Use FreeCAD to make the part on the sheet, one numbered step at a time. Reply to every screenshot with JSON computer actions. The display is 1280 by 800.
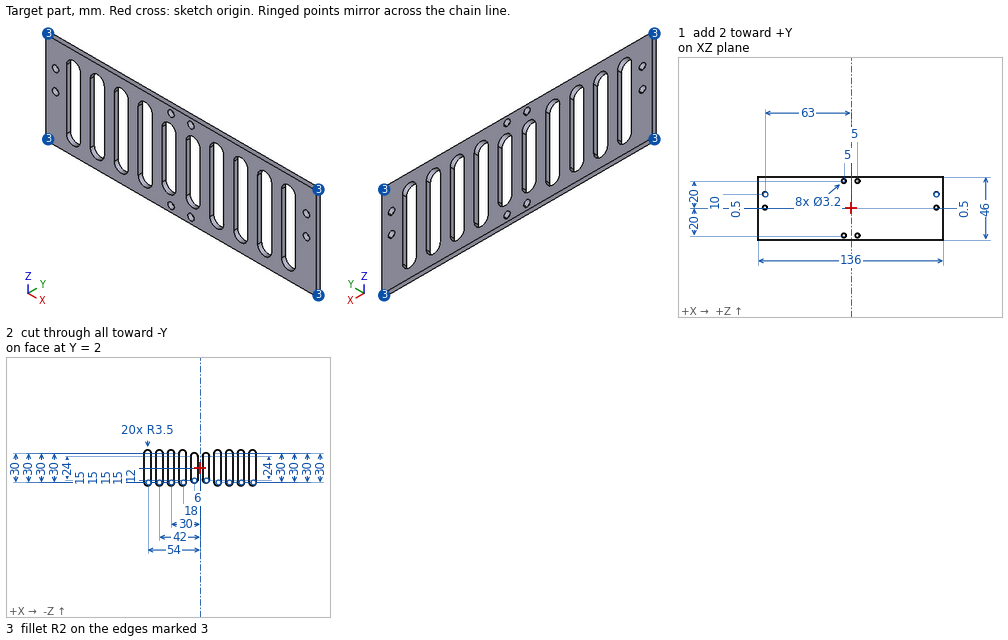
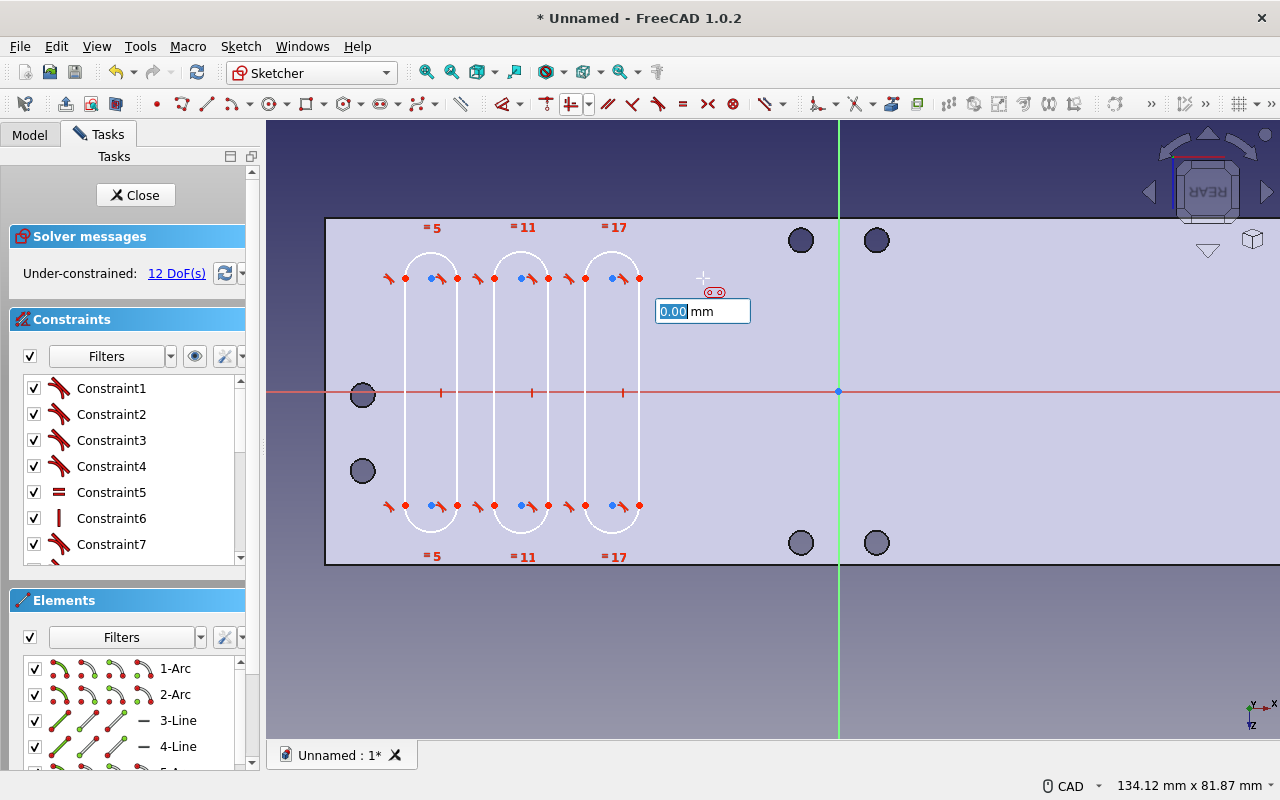
{"action": "left_click", "coordinate": [729, 426]}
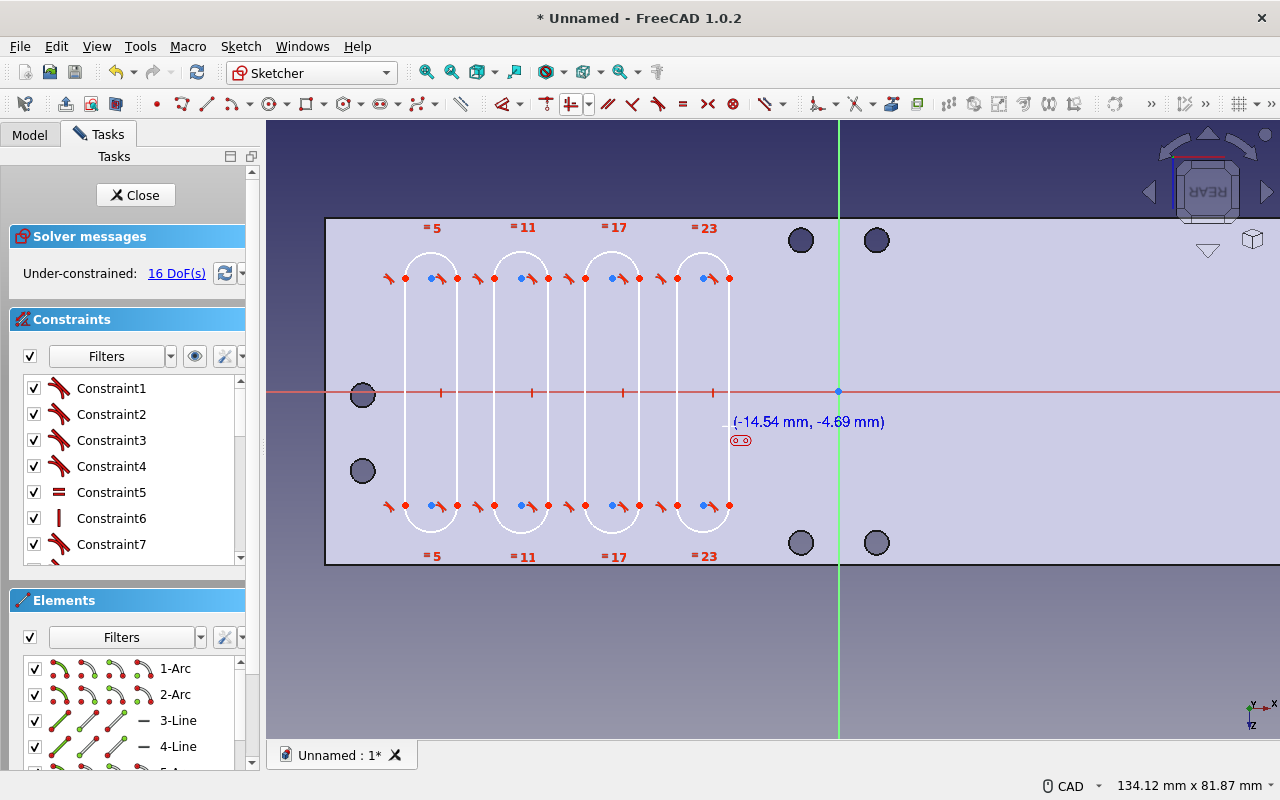
{"action": "left_click", "coordinate": [794, 482]}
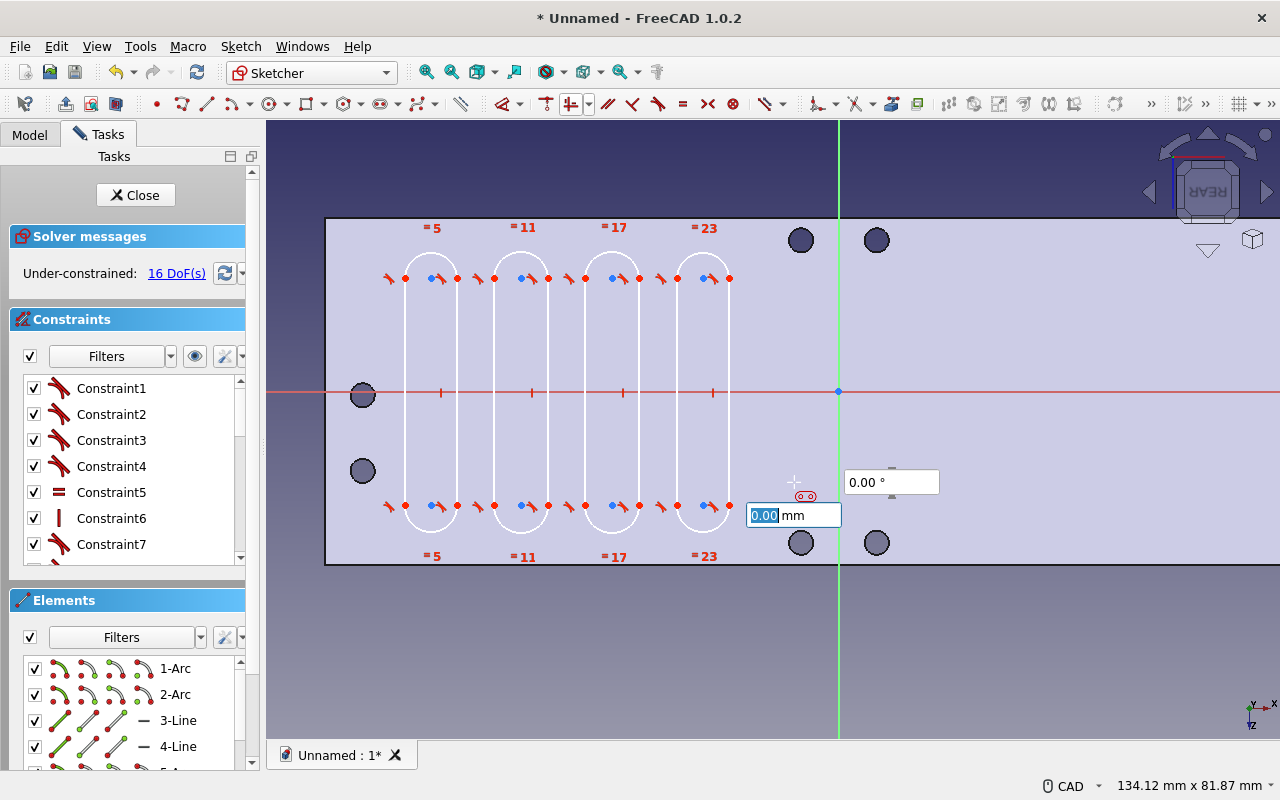
{"action": "left_click", "coordinate": [794, 301]}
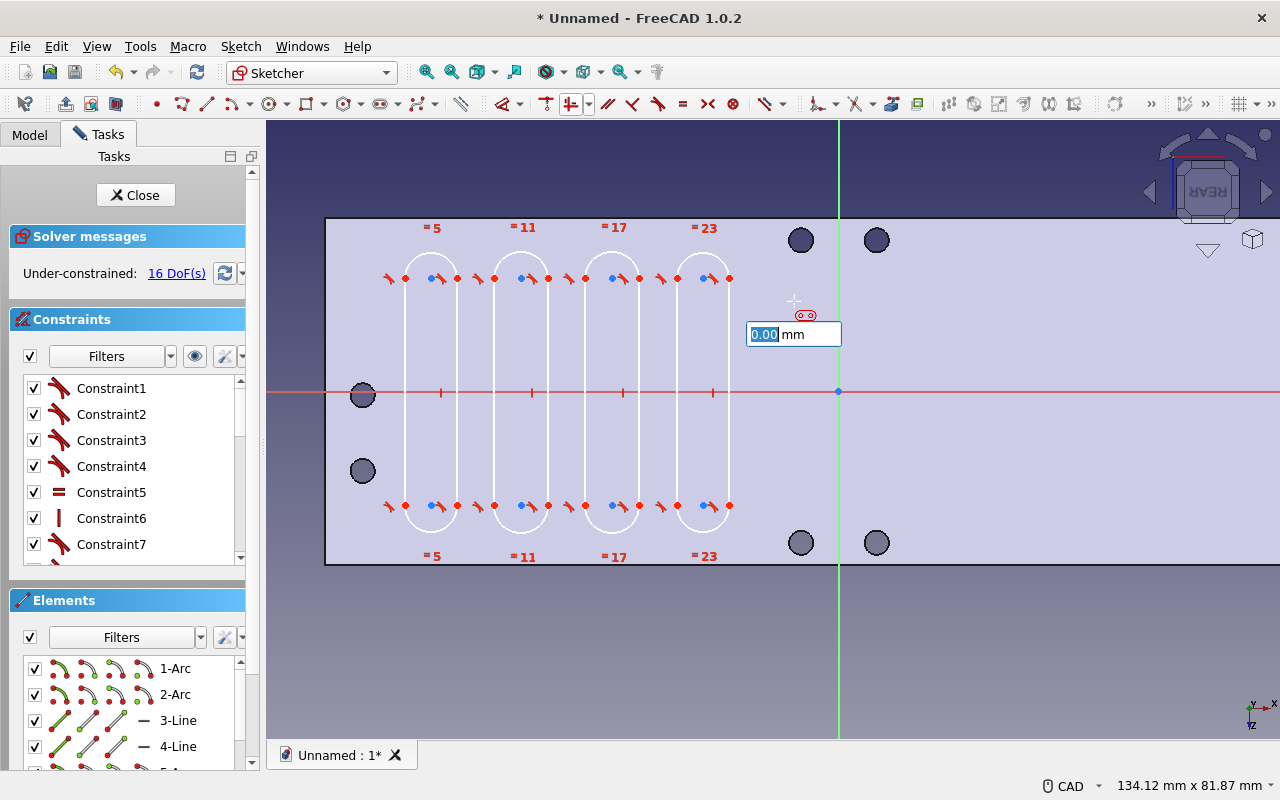
{"action": "left_click", "coordinate": [820, 419]}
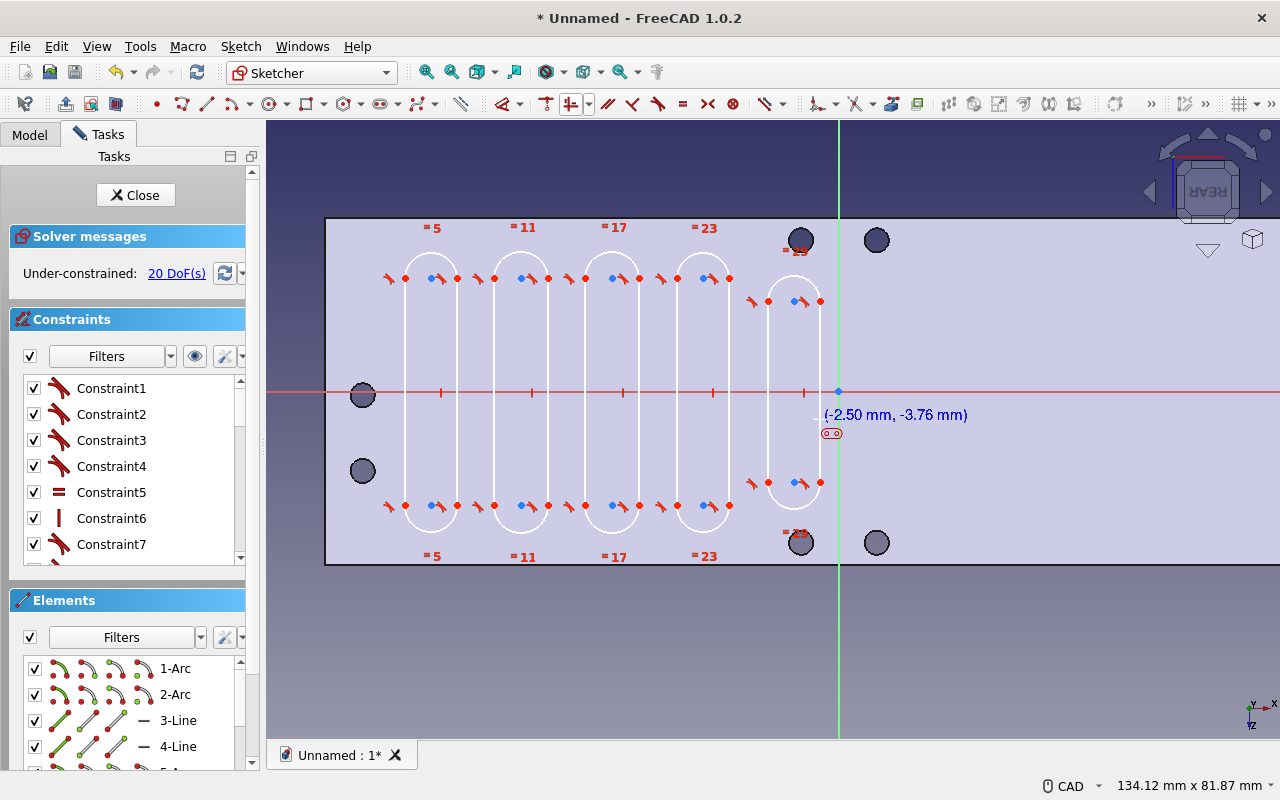
{"action": "left_click", "coordinate": [884, 482]}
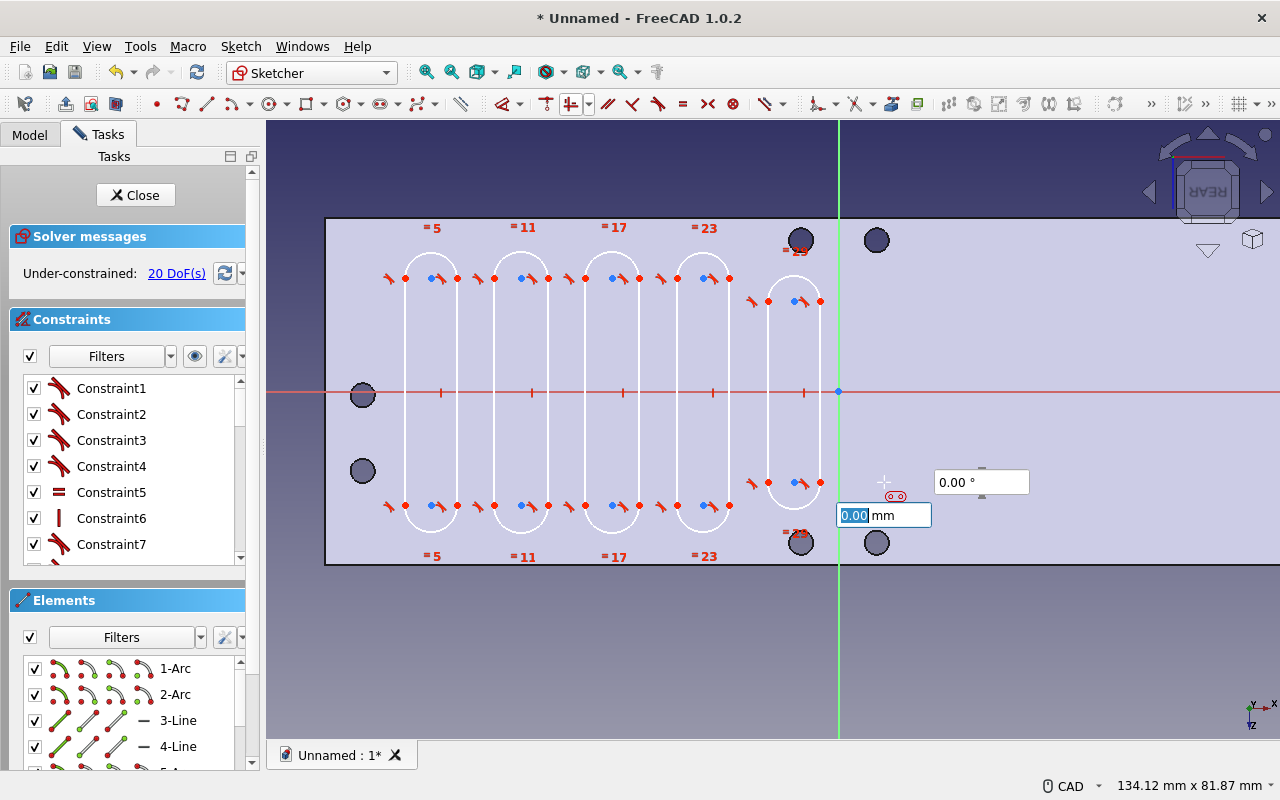
{"action": "left_click", "coordinate": [884, 301]}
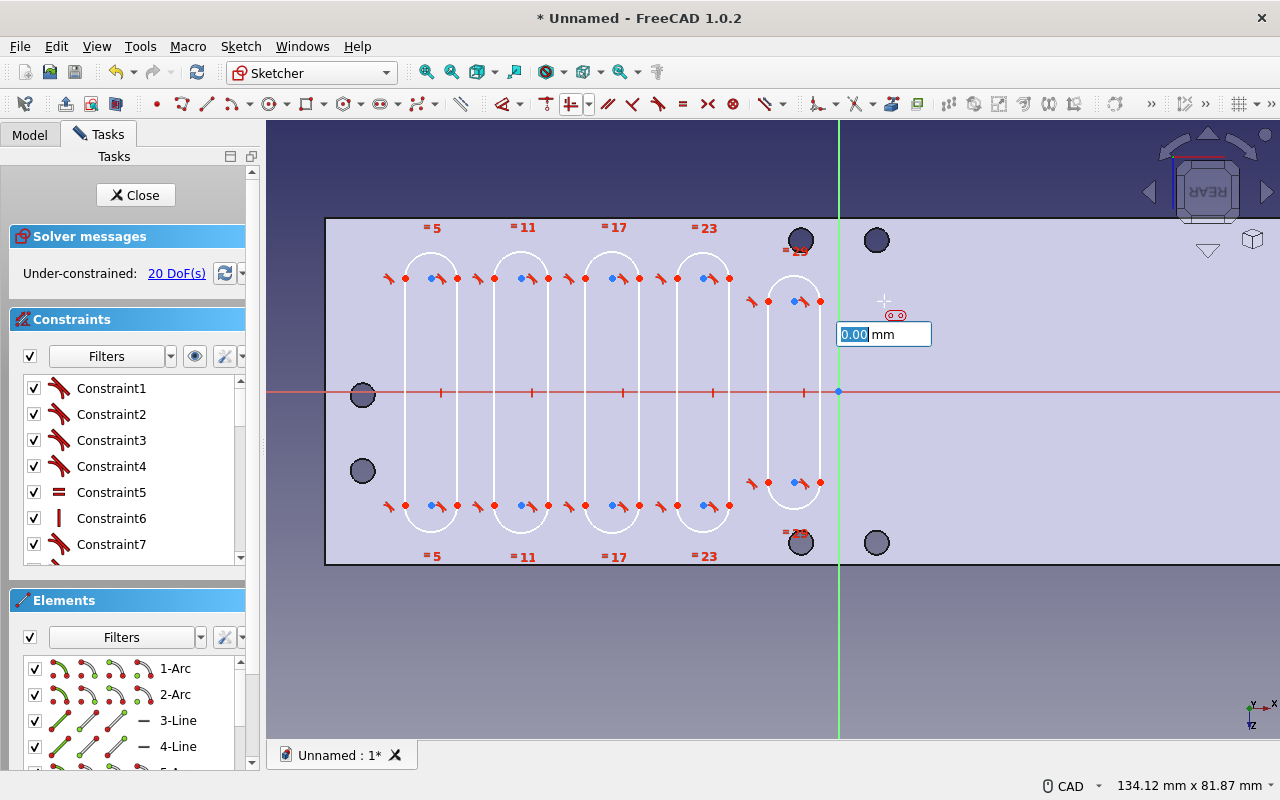
{"action": "left_click", "coordinate": [911, 419]}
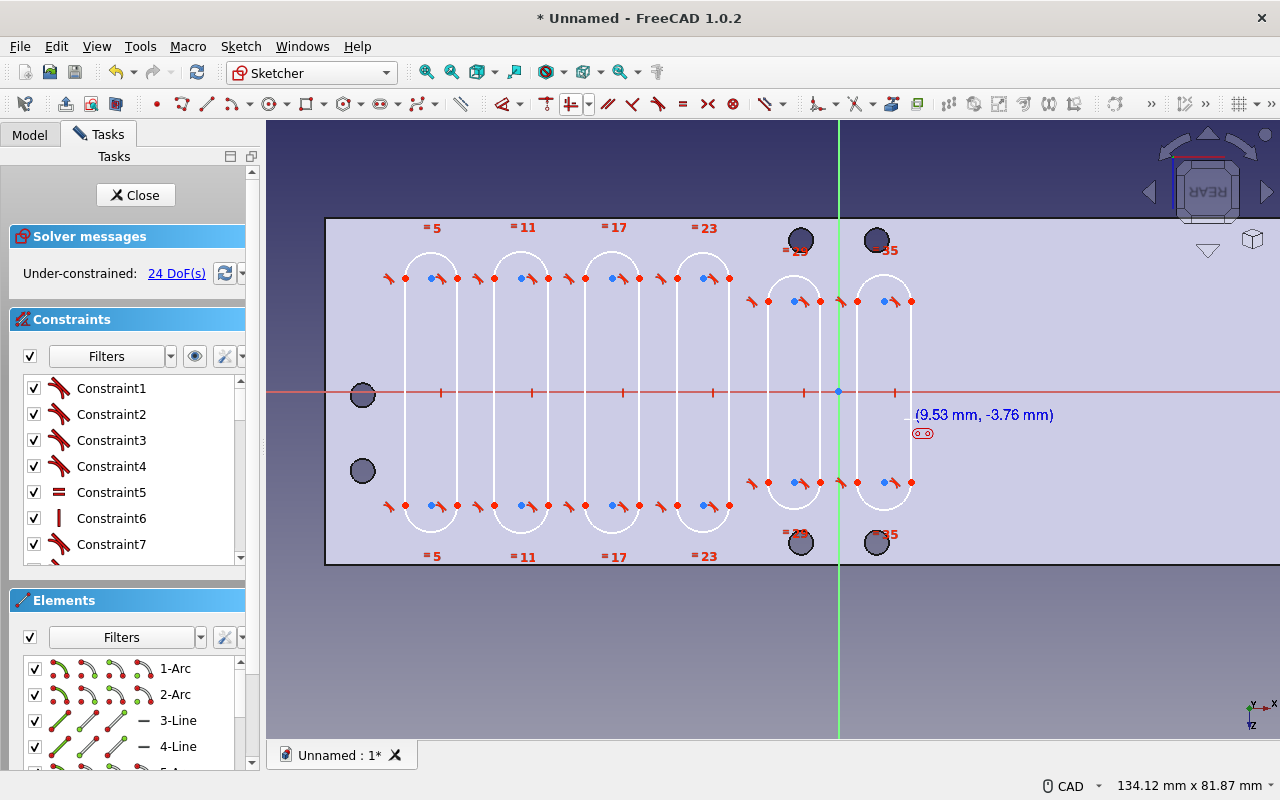
{"action": "left_click", "coordinate": [975, 505]}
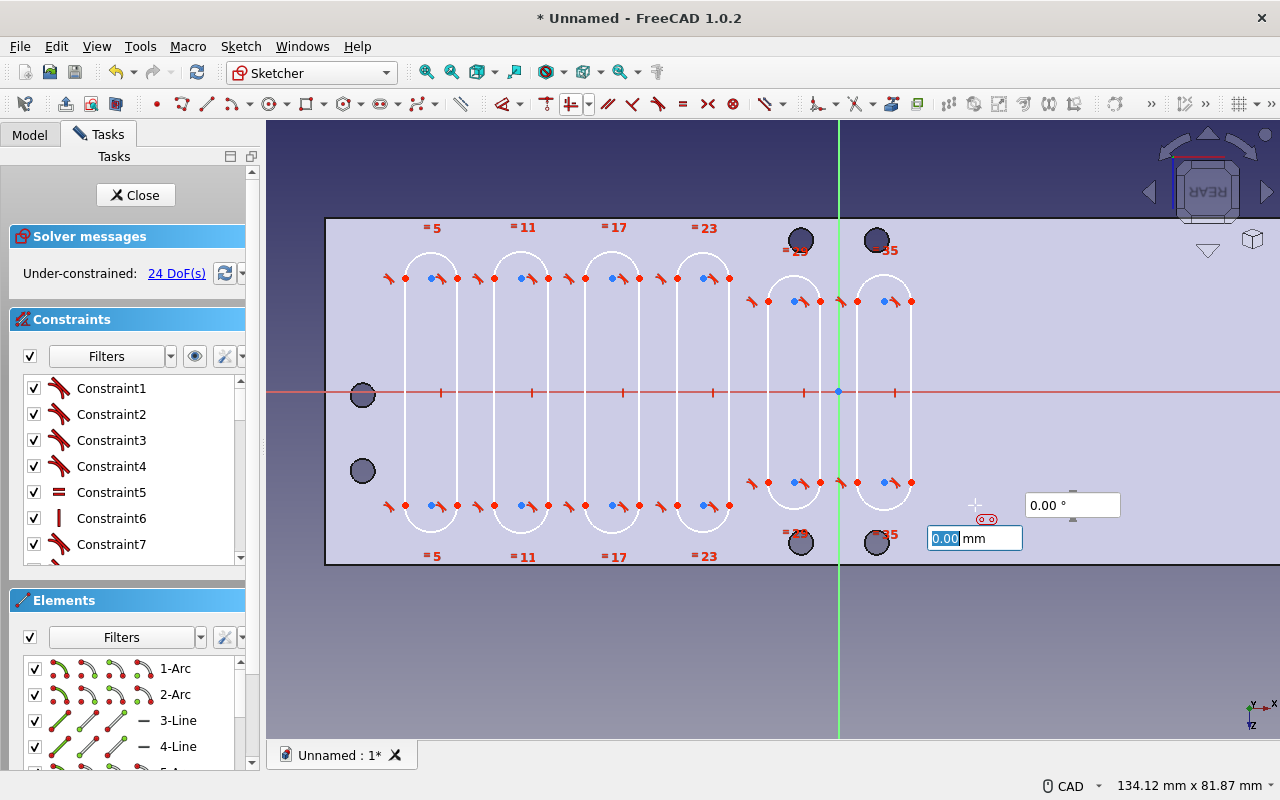
{"action": "left_click", "coordinate": [975, 278]}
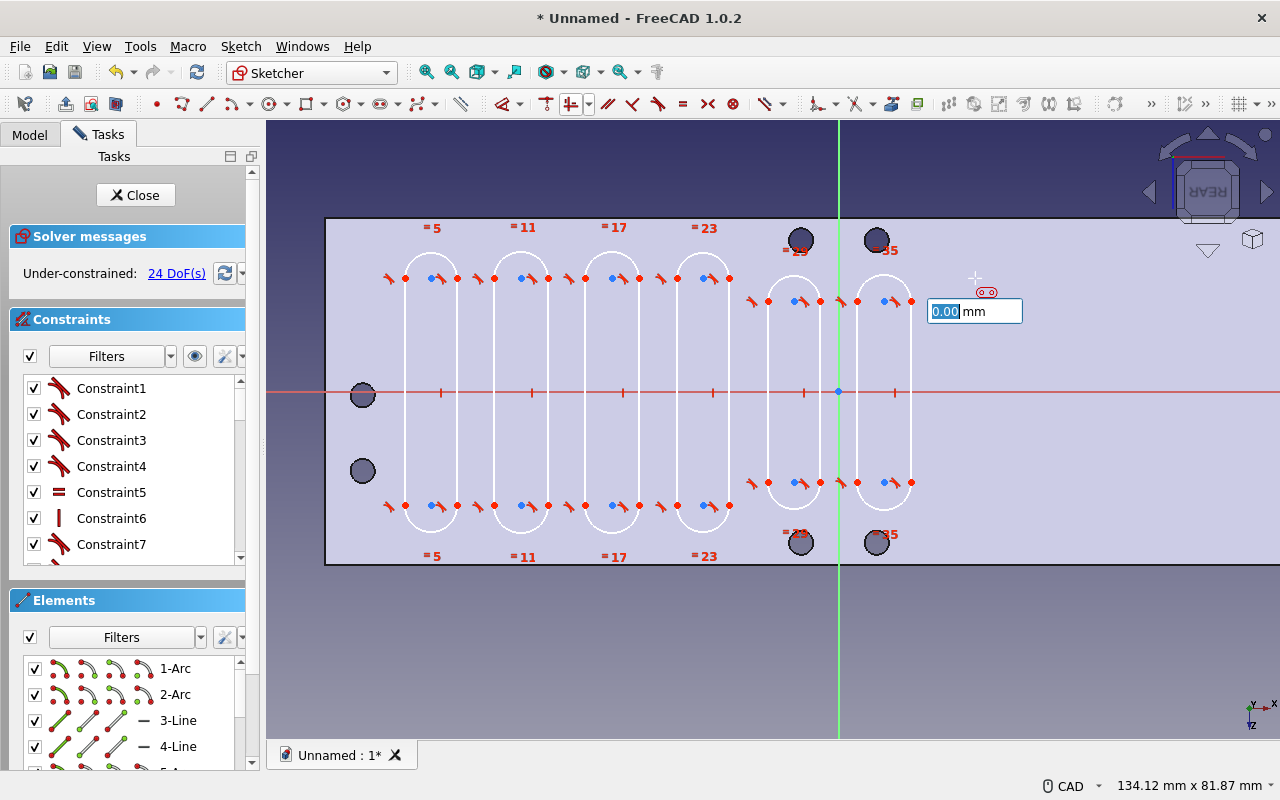
{"action": "left_click", "coordinate": [1001, 426]}